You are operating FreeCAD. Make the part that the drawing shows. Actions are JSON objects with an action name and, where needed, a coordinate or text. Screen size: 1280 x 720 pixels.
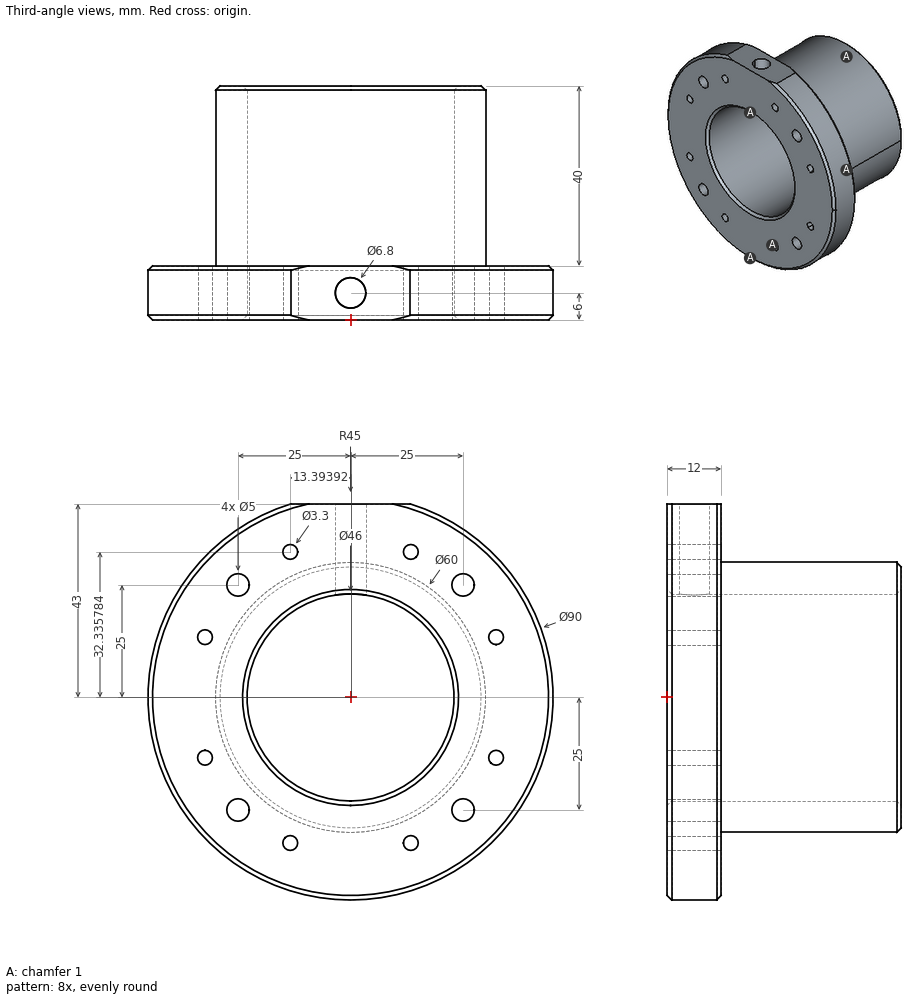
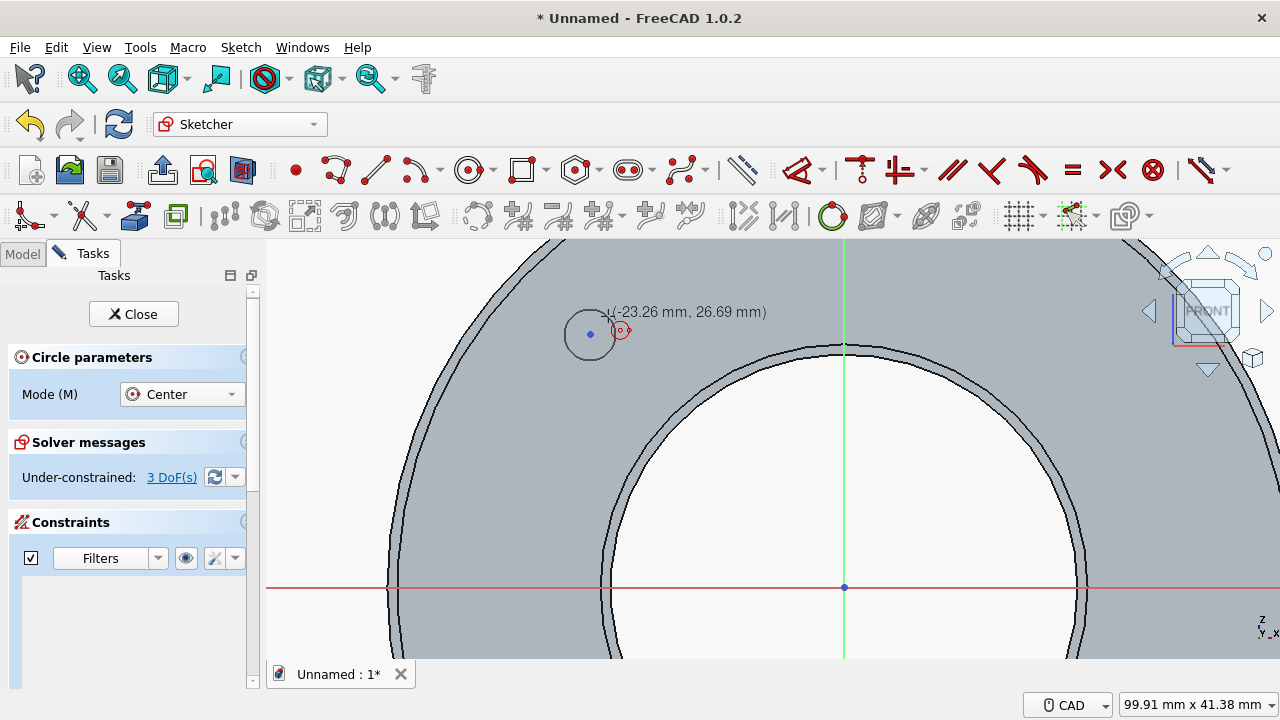
{"action": "left_click", "coordinate": [1098, 334]}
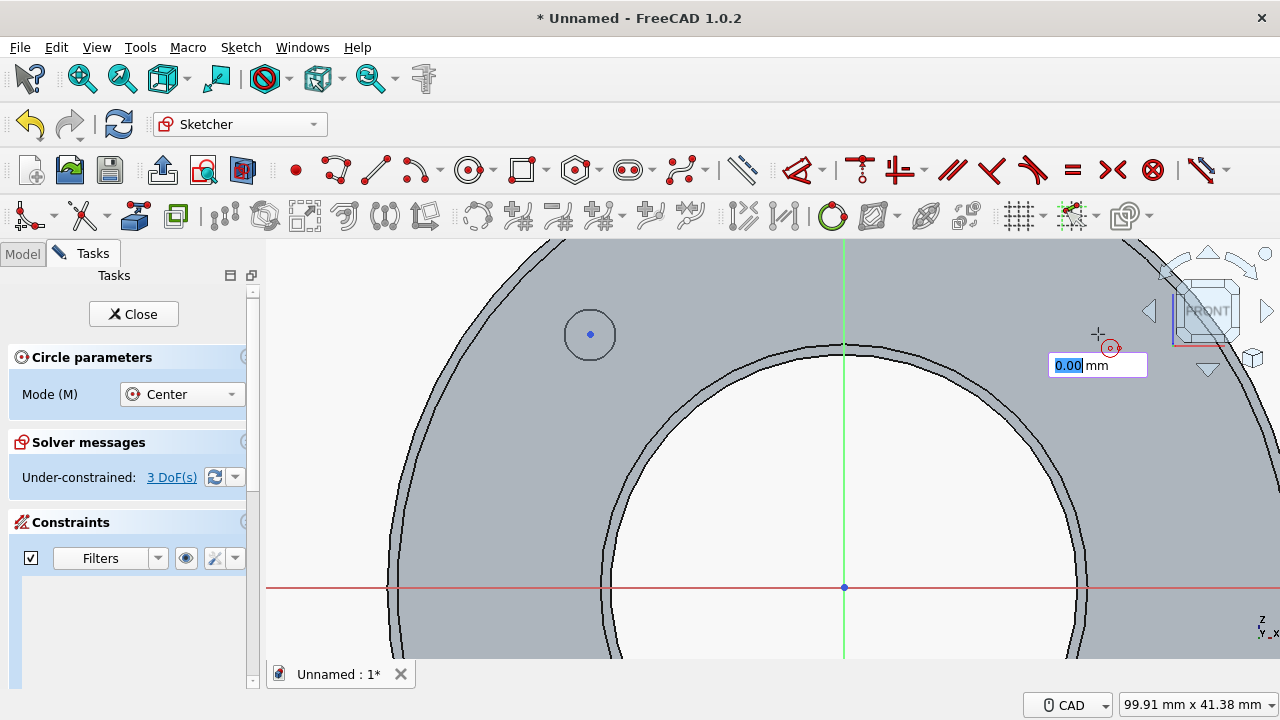
{"action": "scroll", "coordinate": [591, 336], "scroll_direction": "down", "scroll_amount": 4}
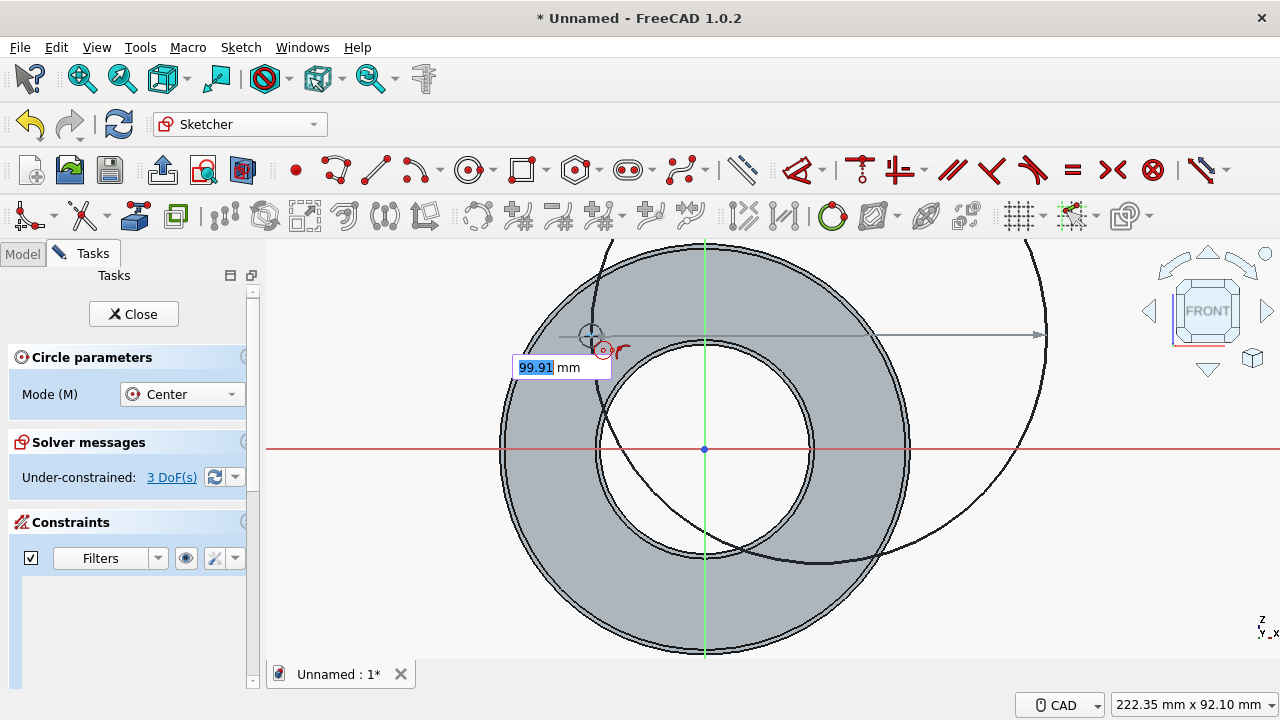
{"action": "scroll", "coordinate": [827, 327], "scroll_direction": "up", "scroll_amount": 2}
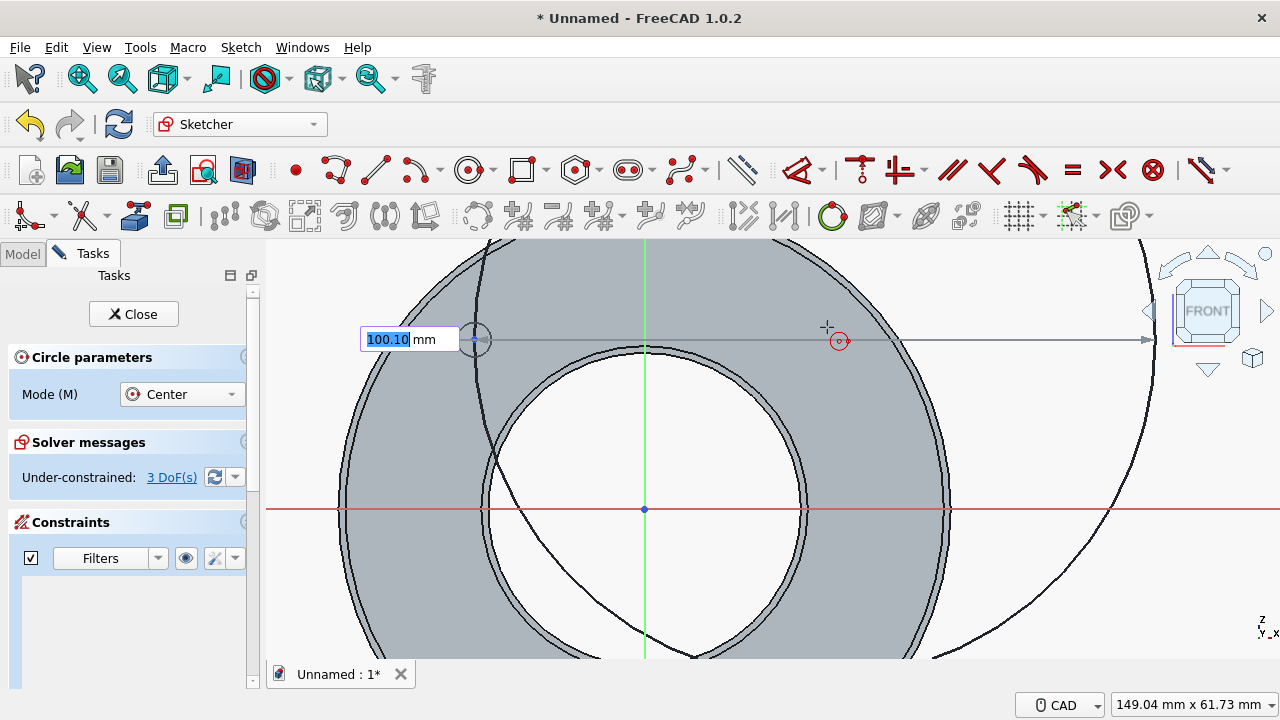
{"action": "left_click", "coordinate": [827, 327]}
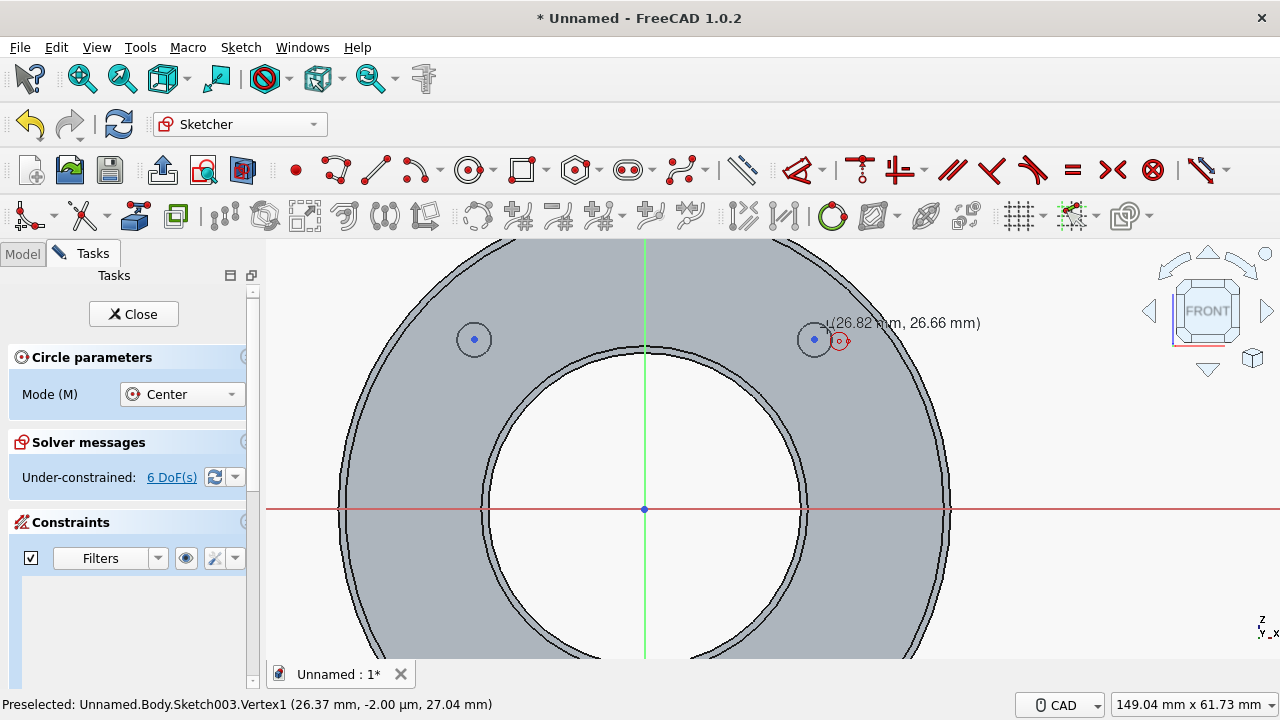
{"action": "scroll", "coordinate": [826, 326], "scroll_direction": "down", "scroll_amount": 2}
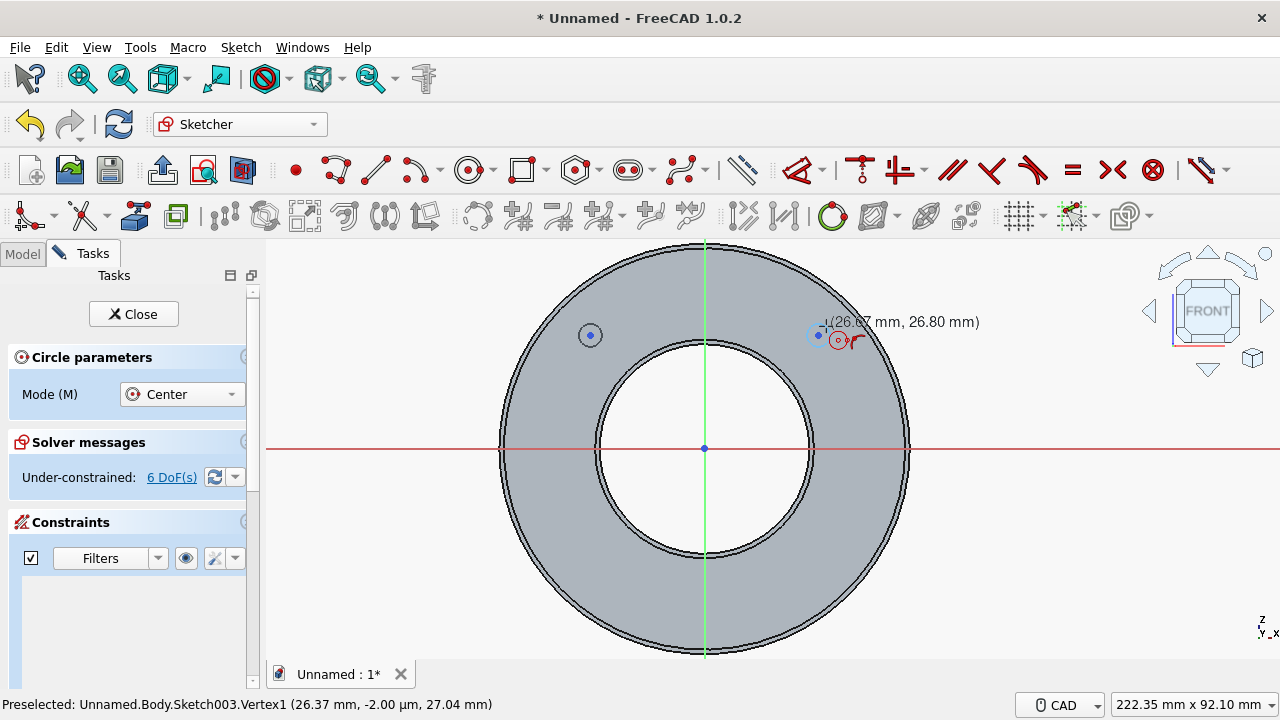
{"action": "scroll", "coordinate": [819, 563], "scroll_direction": "up", "scroll_amount": 4}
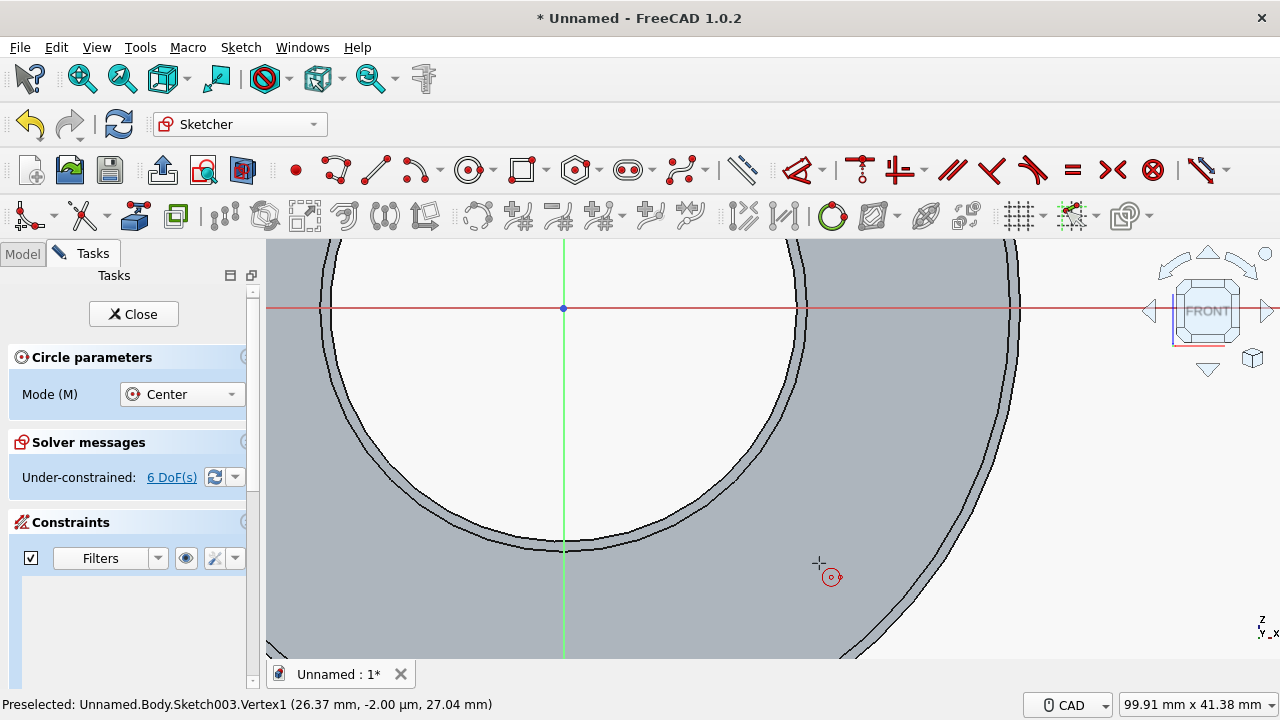
{"action": "left_click", "coordinate": [817, 562]}
{"action": "left_click", "coordinate": [835, 544]}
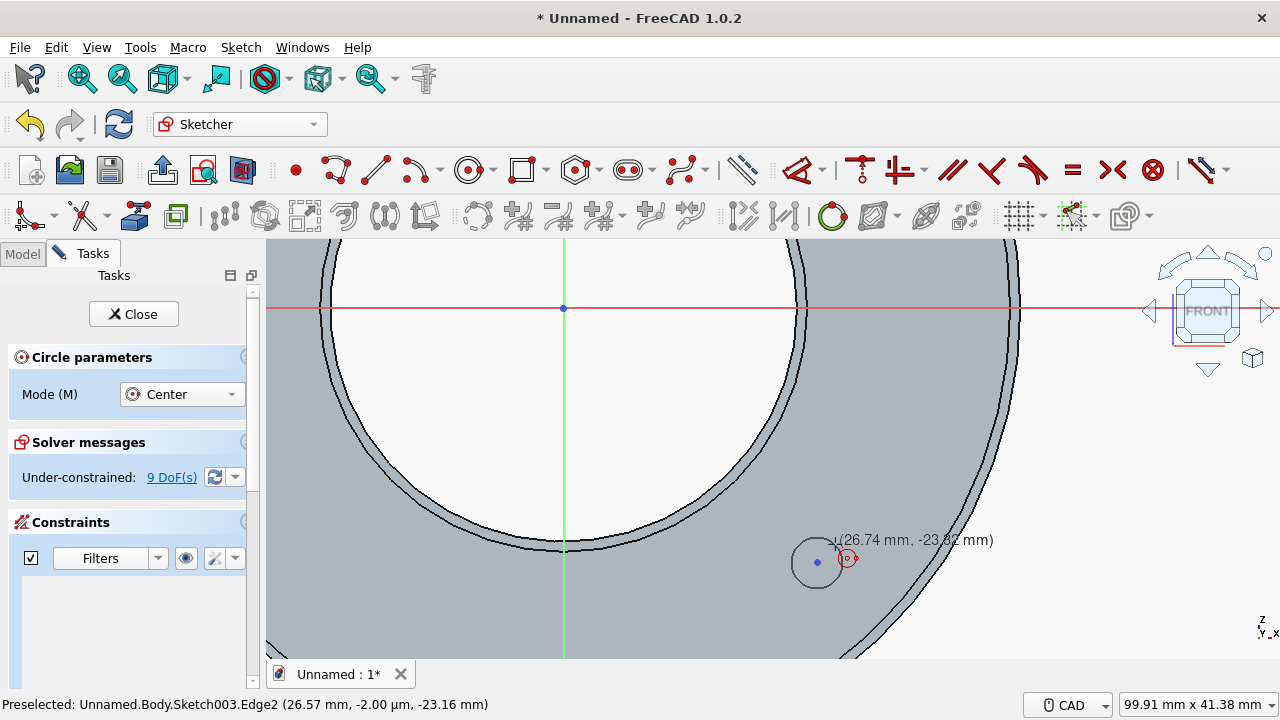
{"action": "left_click", "coordinate": [310, 562]}
{"action": "left_click", "coordinate": [328, 544]}
{"action": "key", "text": "Escape"}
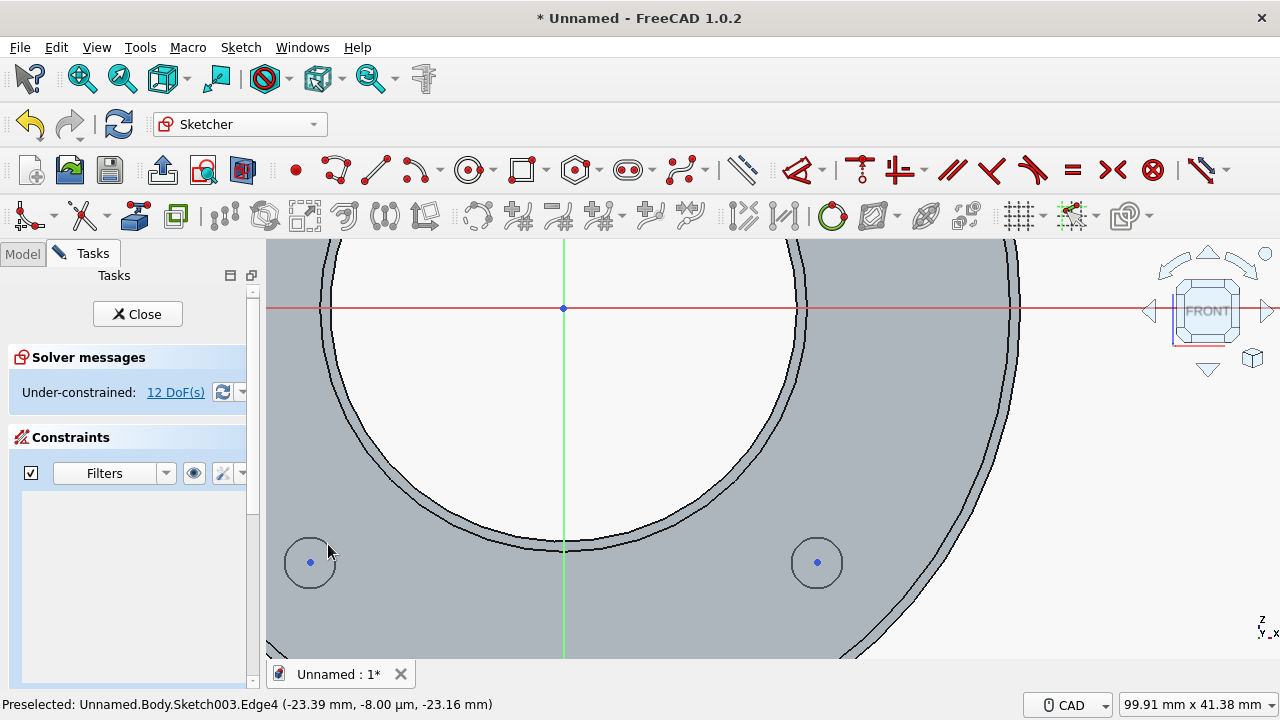
{"action": "scroll", "coordinate": [819, 564], "scroll_direction": "down", "scroll_amount": 4}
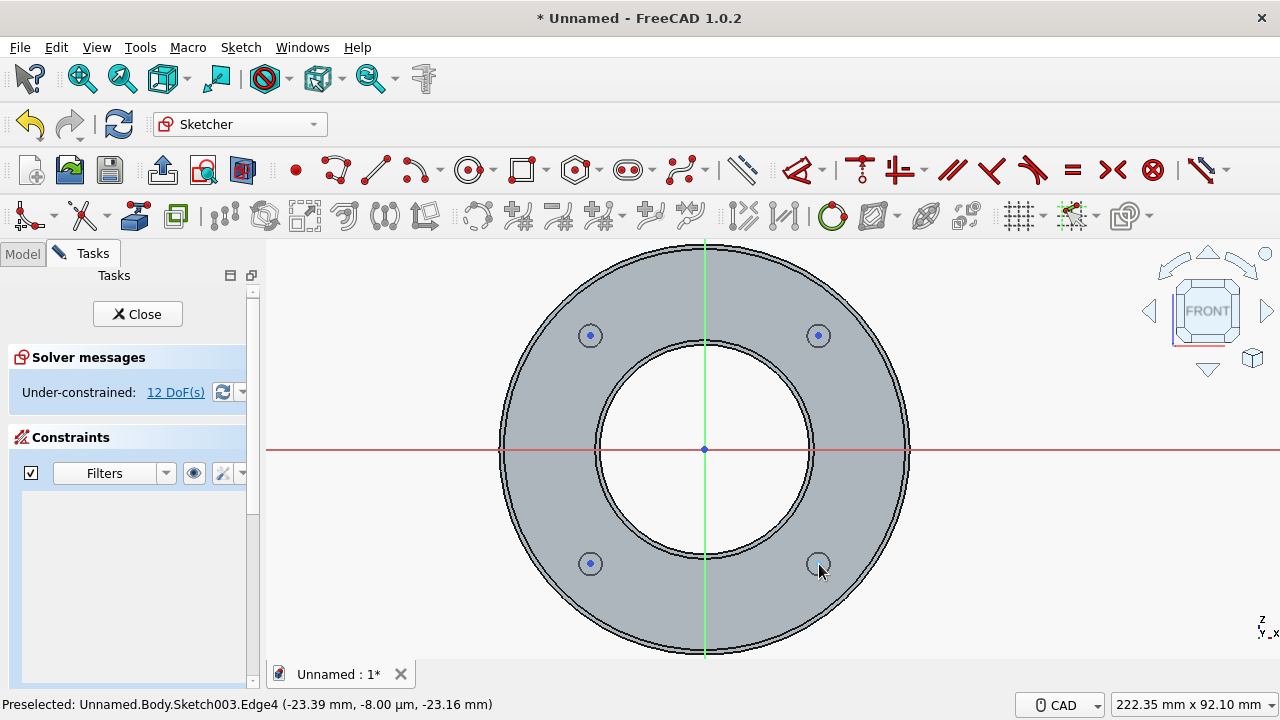
{"action": "left_click", "coordinate": [598, 328]}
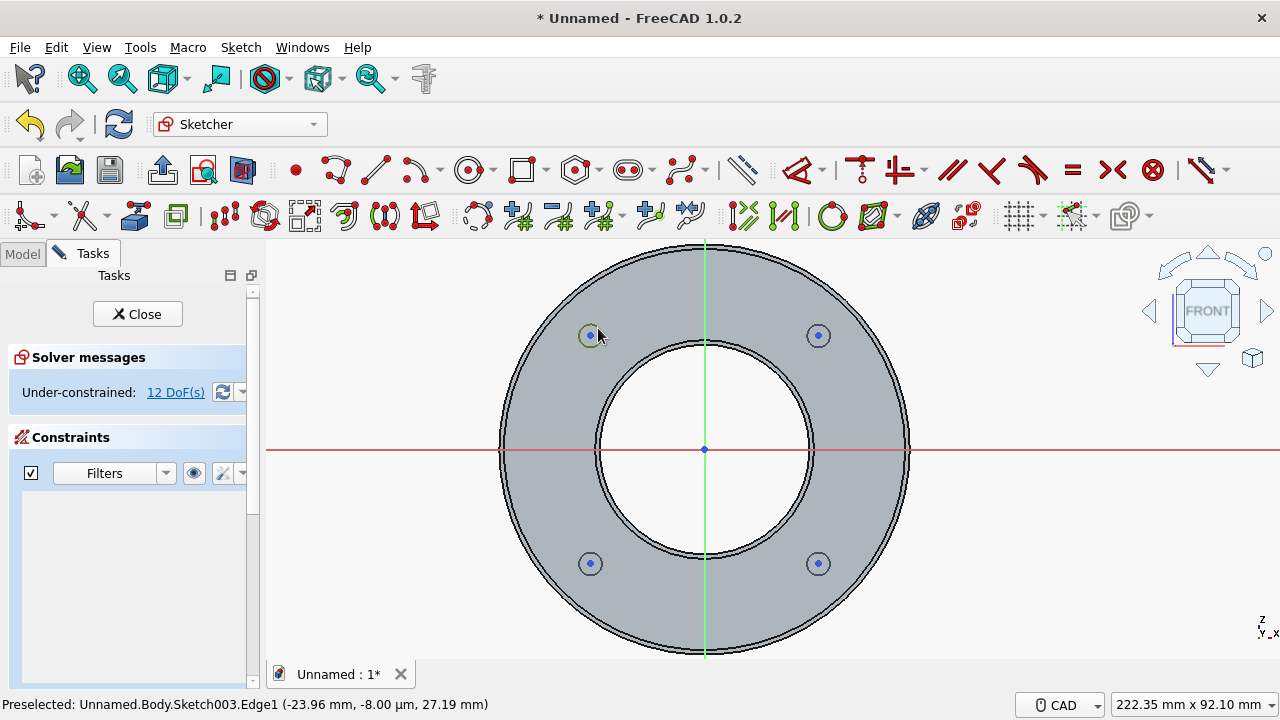
{"action": "left_click", "coordinate": [827, 328]}